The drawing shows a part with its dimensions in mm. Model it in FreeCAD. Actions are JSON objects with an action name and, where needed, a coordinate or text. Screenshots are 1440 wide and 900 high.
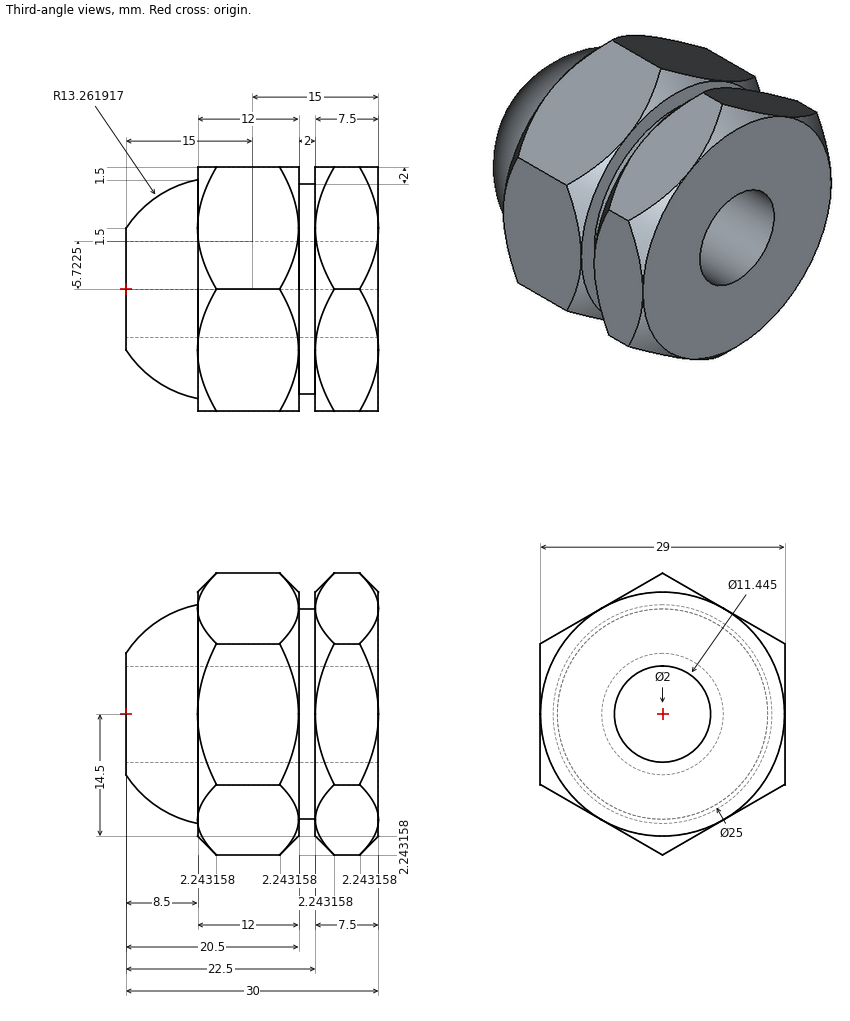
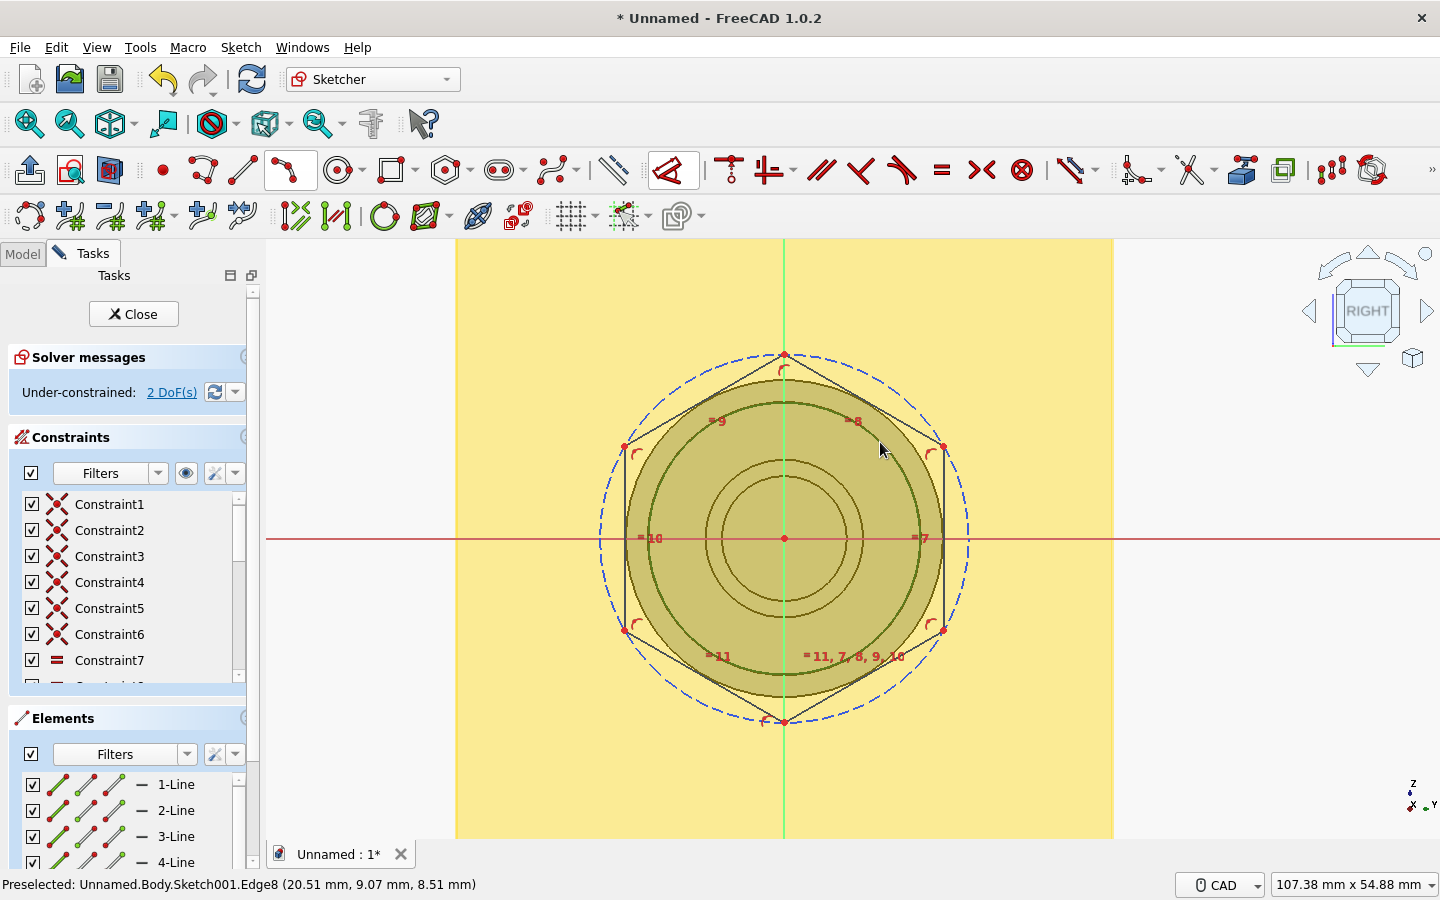
{"action": "left_click", "coordinate": [694, 170]}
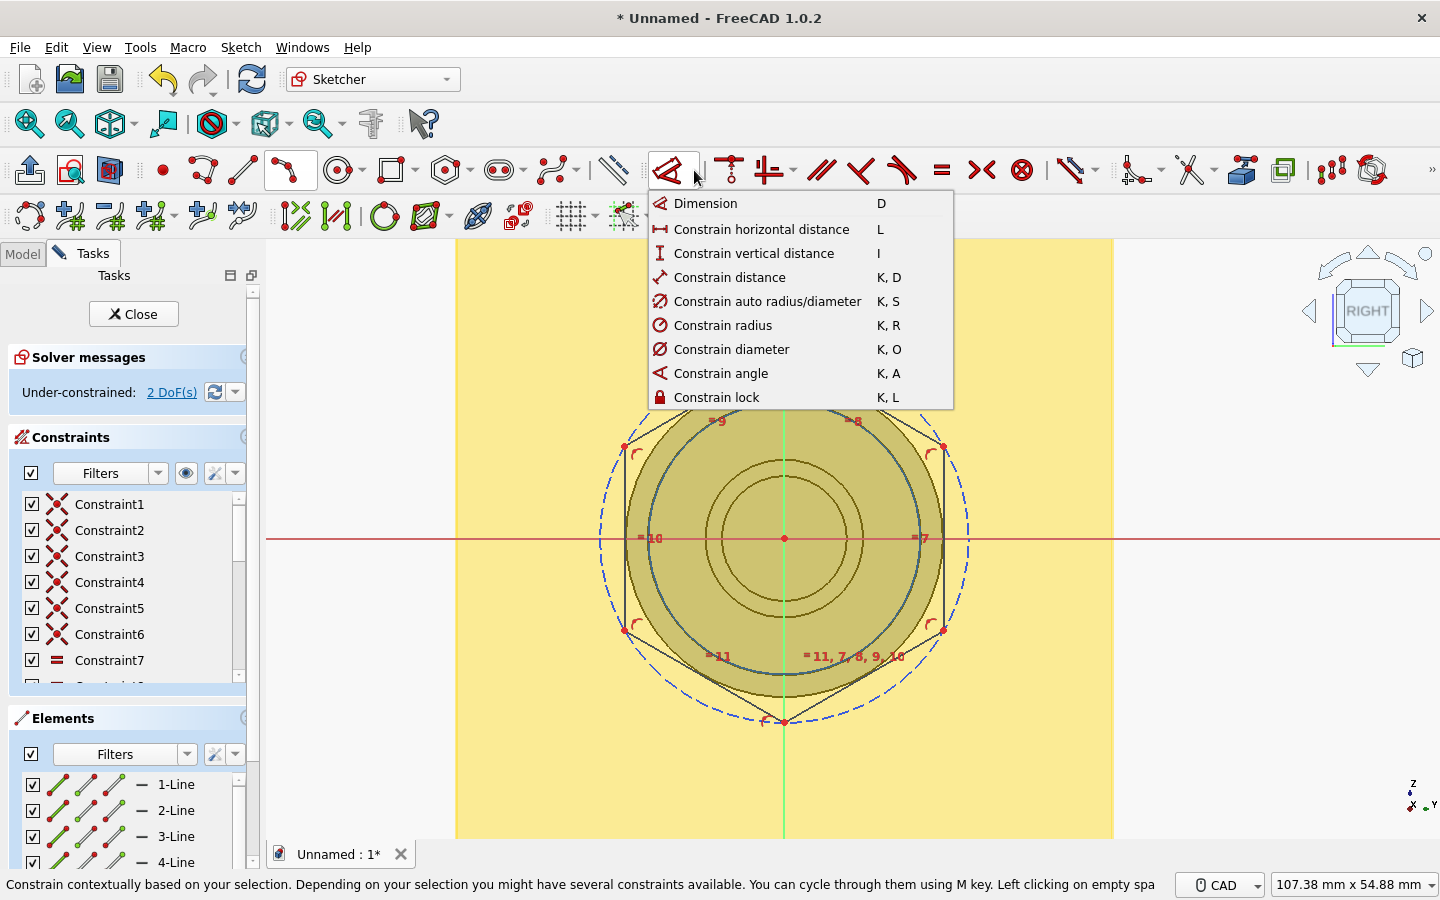
{"action": "left_click", "coordinate": [801, 349]}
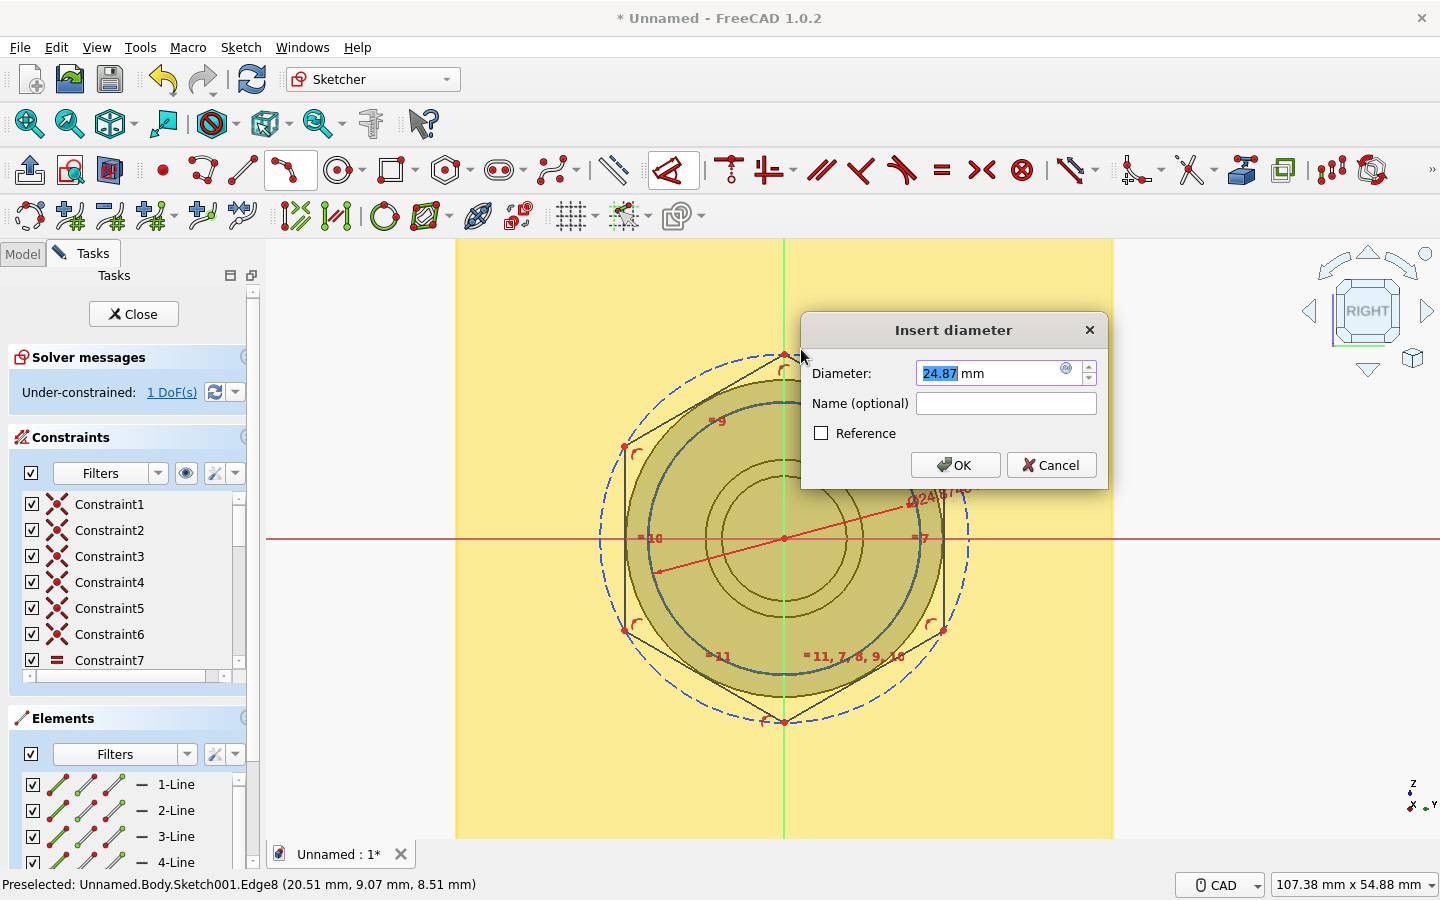
{"action": "type", "text": "25"}
{"action": "key", "text": "Return"}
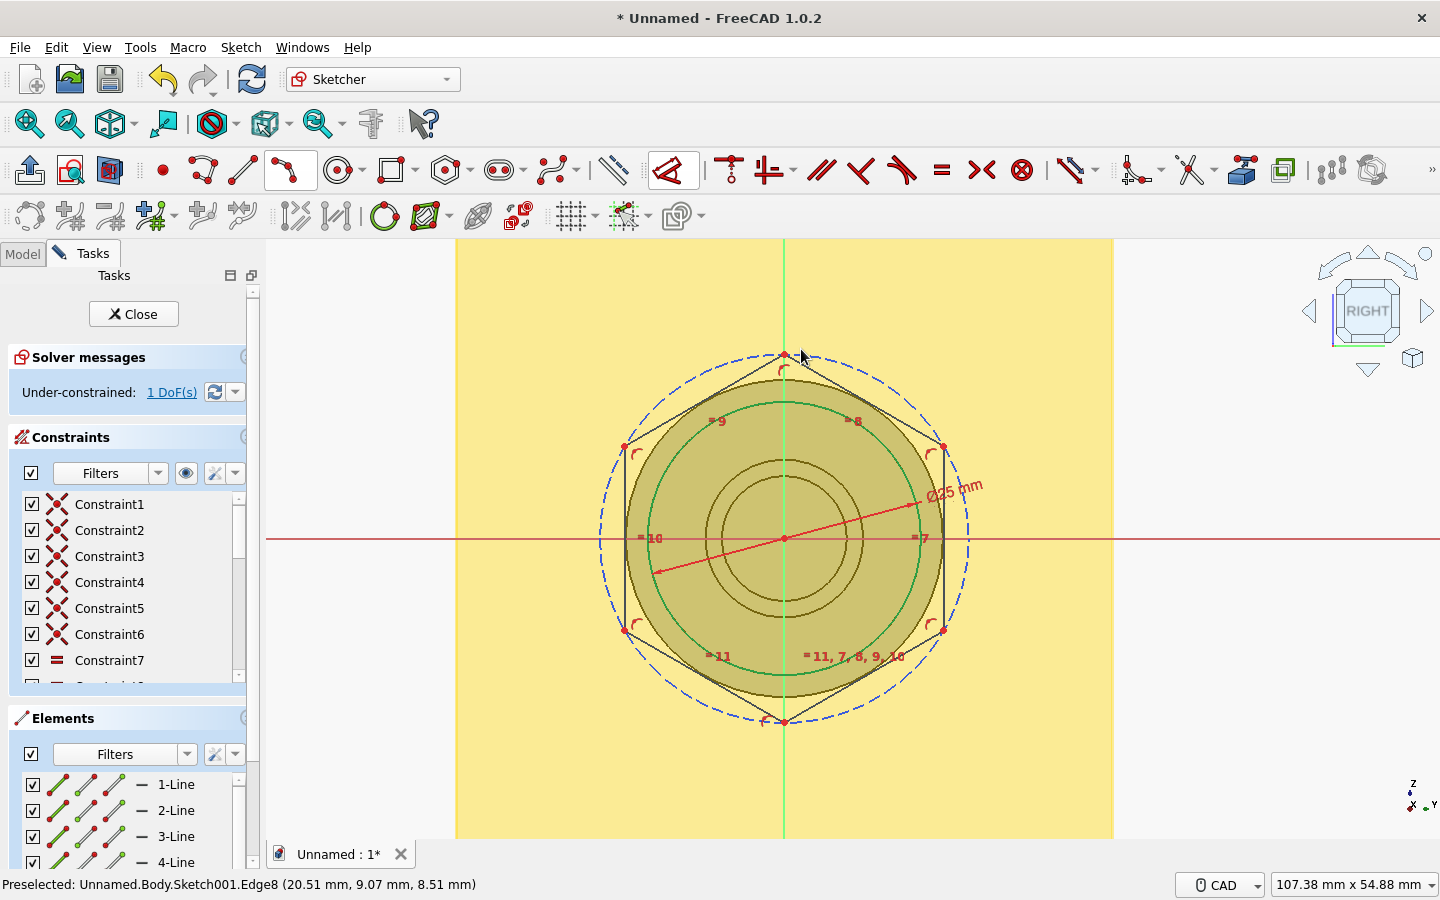
{"action": "left_click", "coordinate": [625, 446]}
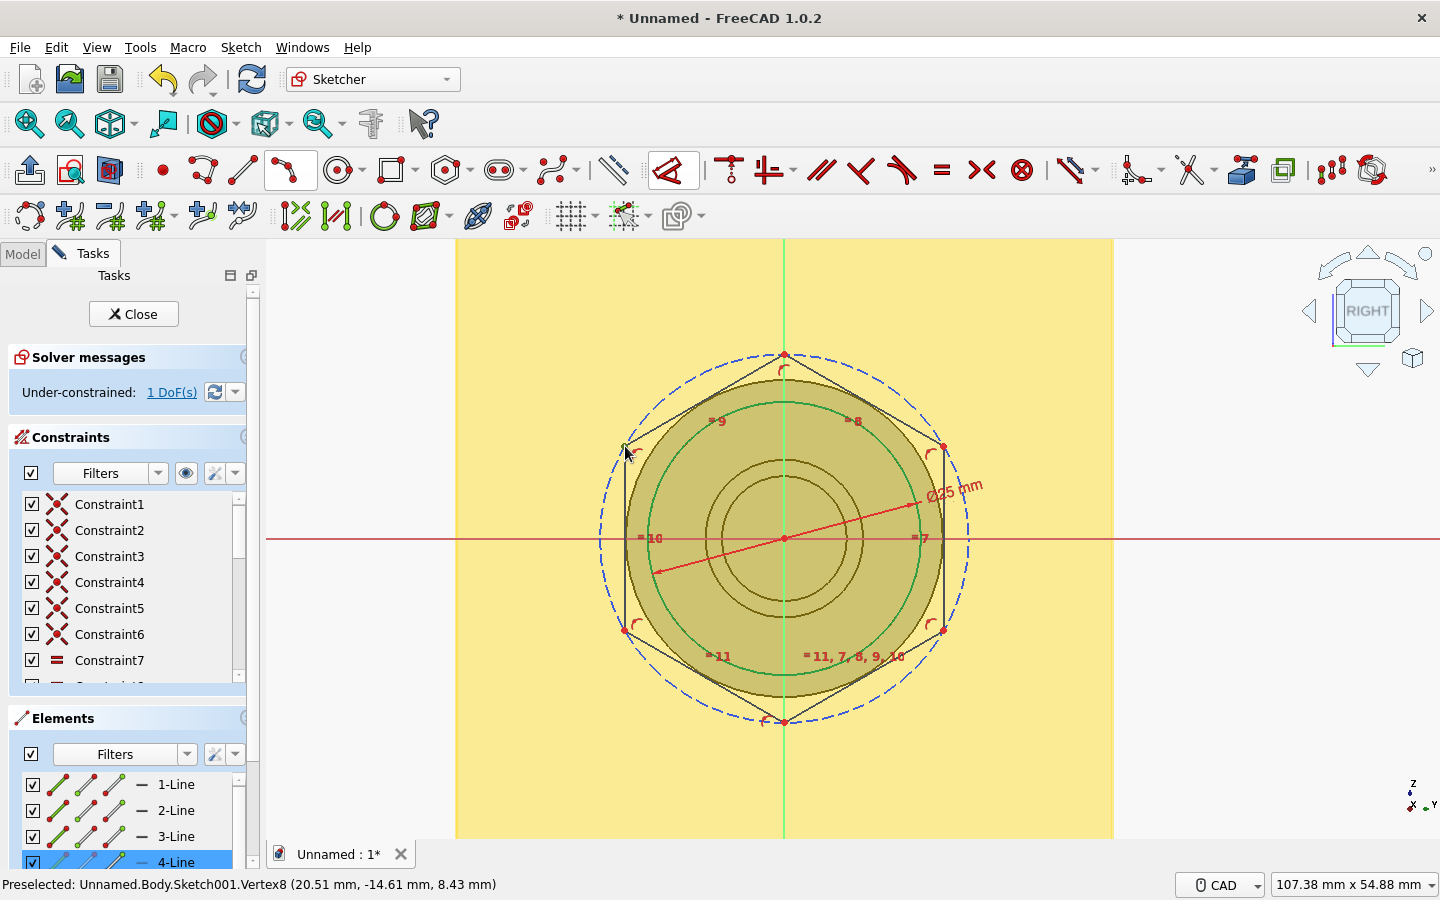
{"action": "left_click", "coordinate": [944, 631]}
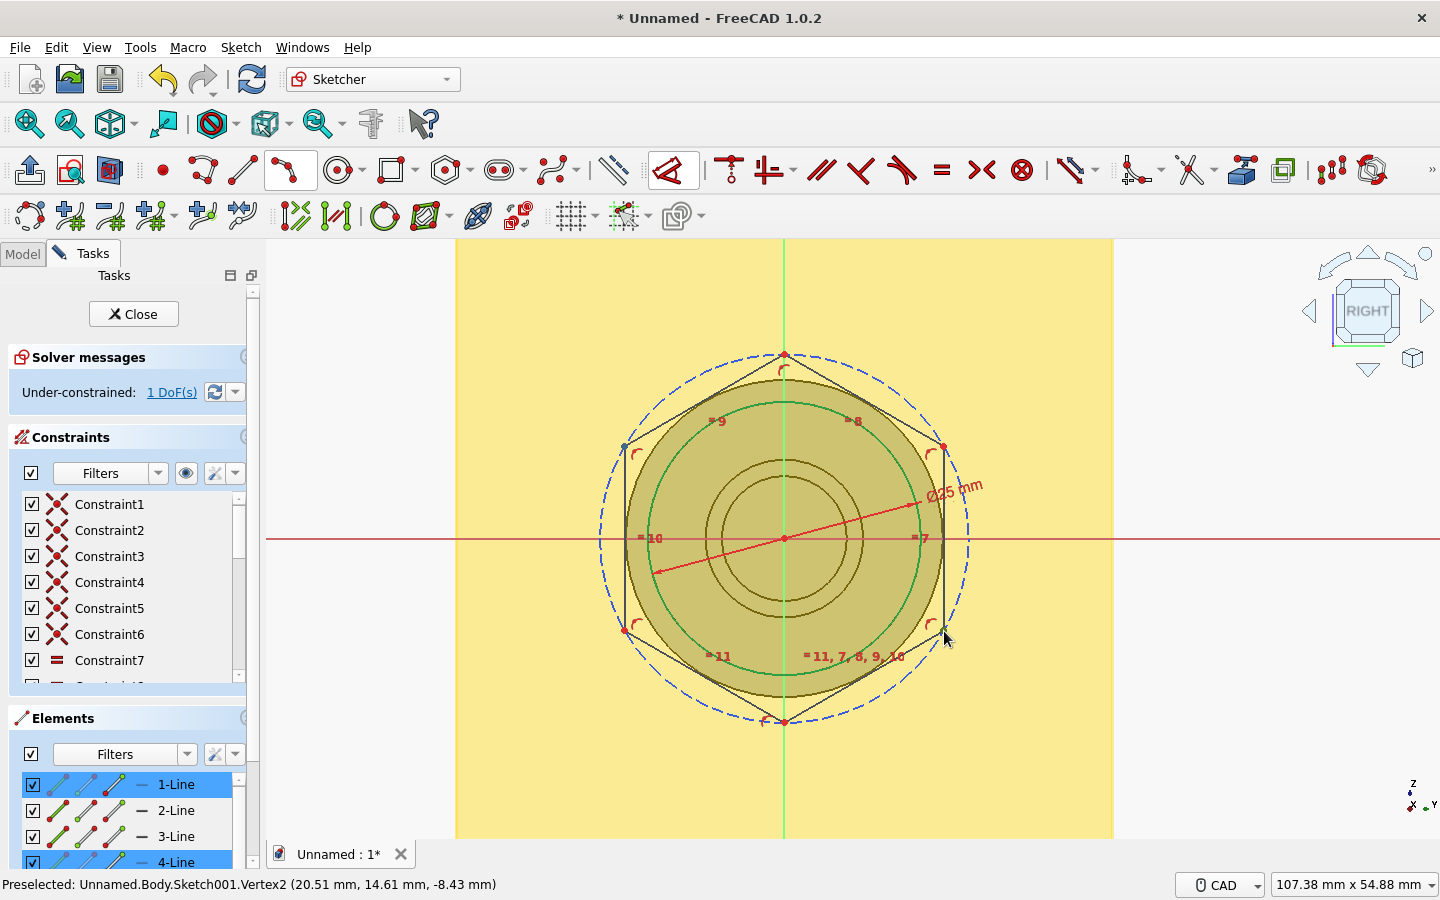
{"action": "key", "text": "l"}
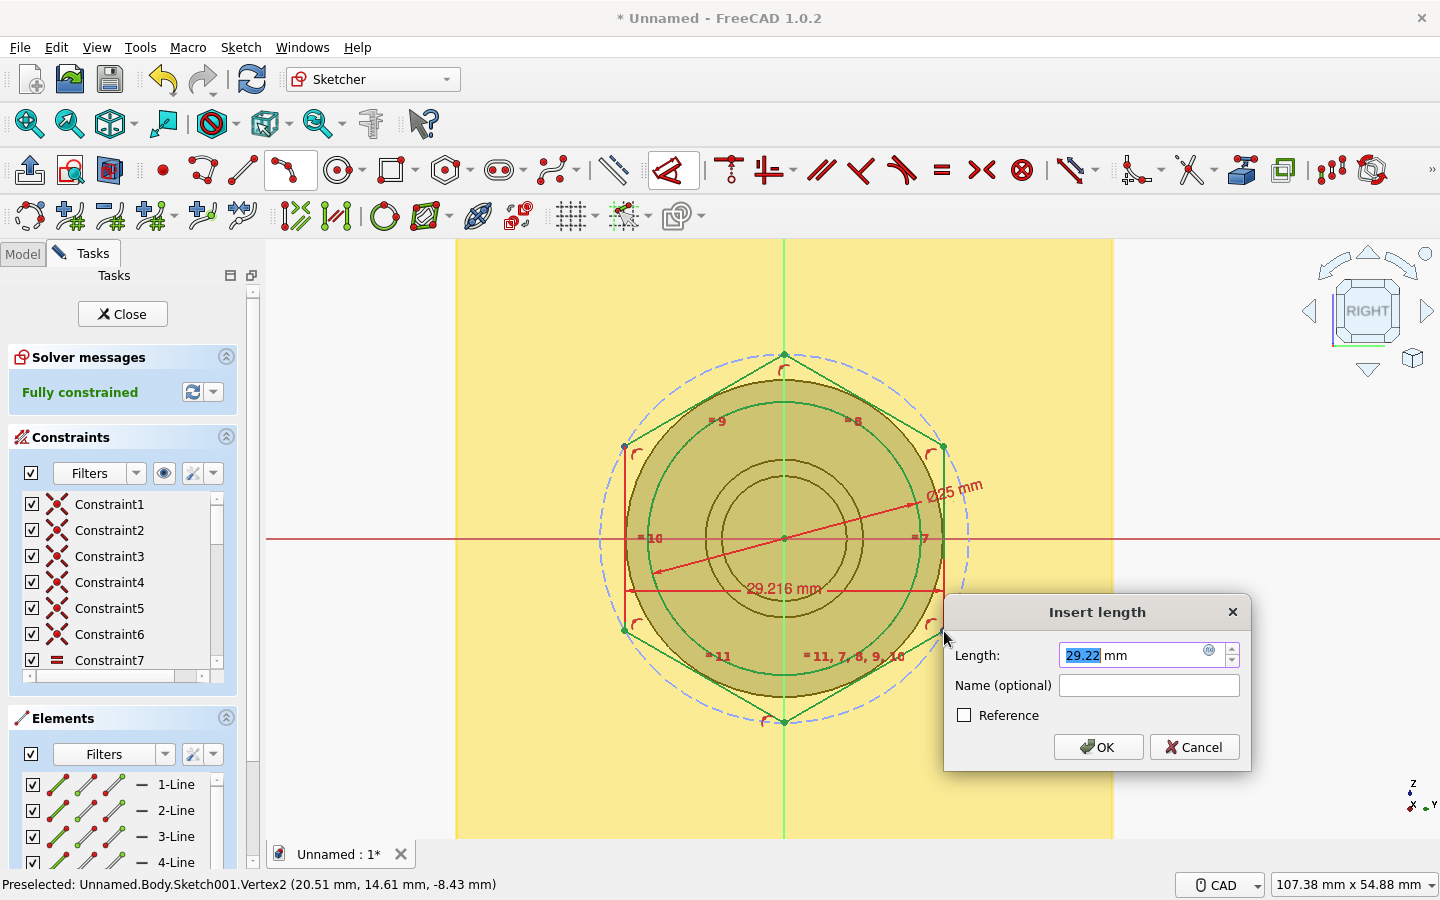
{"action": "type", "text": "29"}
{"action": "key", "text": "Return"}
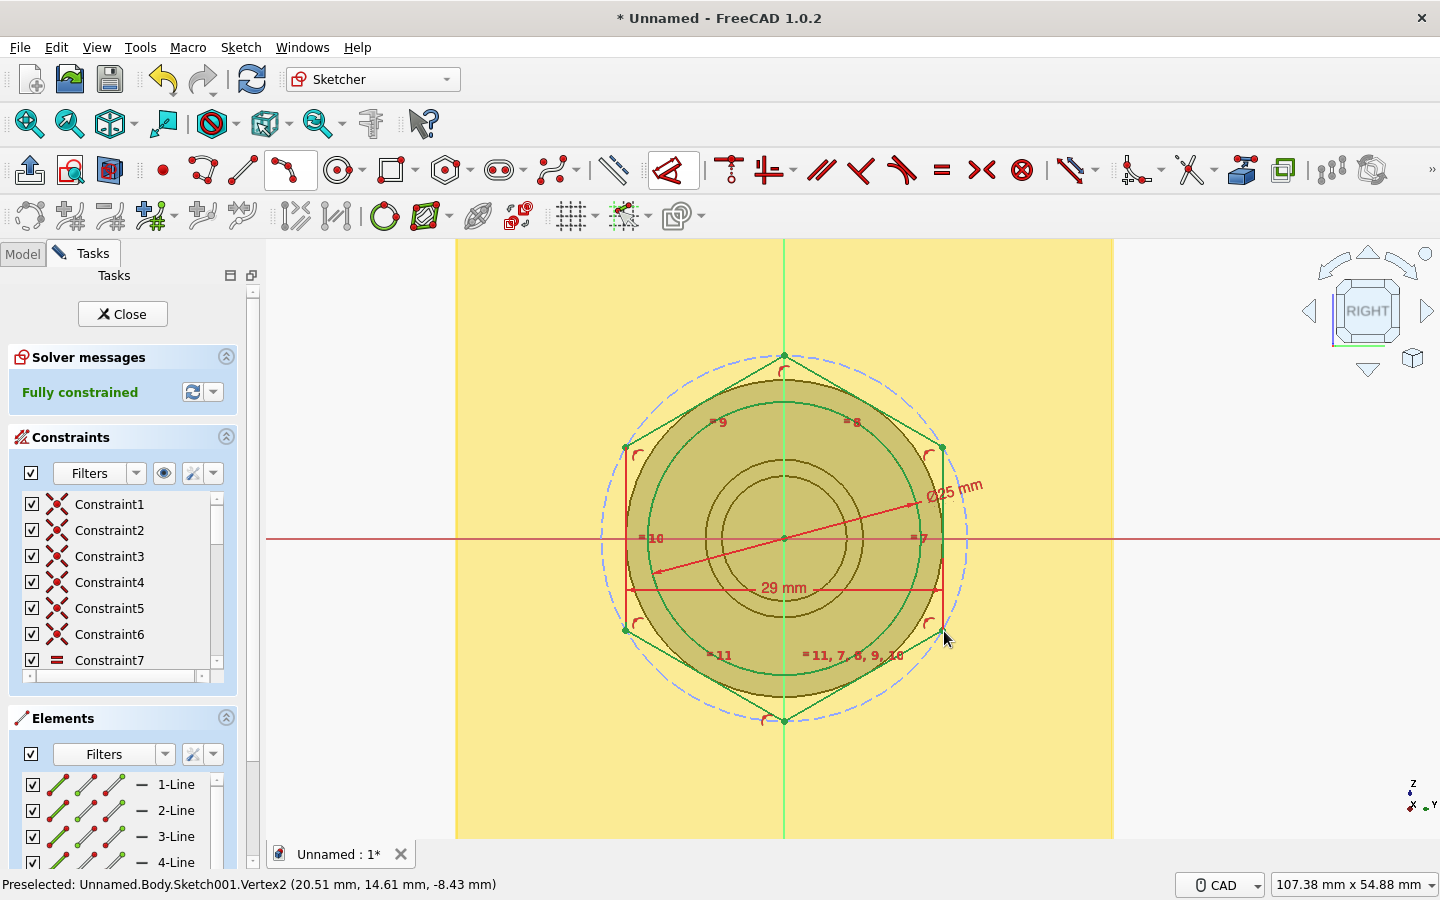
{"action": "left_click", "coordinate": [123, 314]}